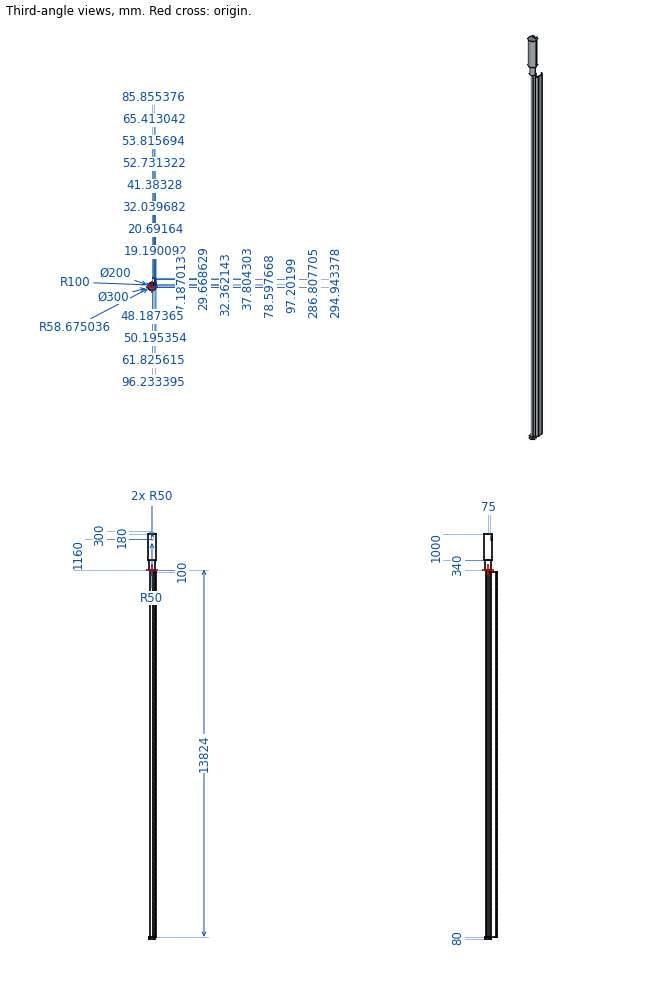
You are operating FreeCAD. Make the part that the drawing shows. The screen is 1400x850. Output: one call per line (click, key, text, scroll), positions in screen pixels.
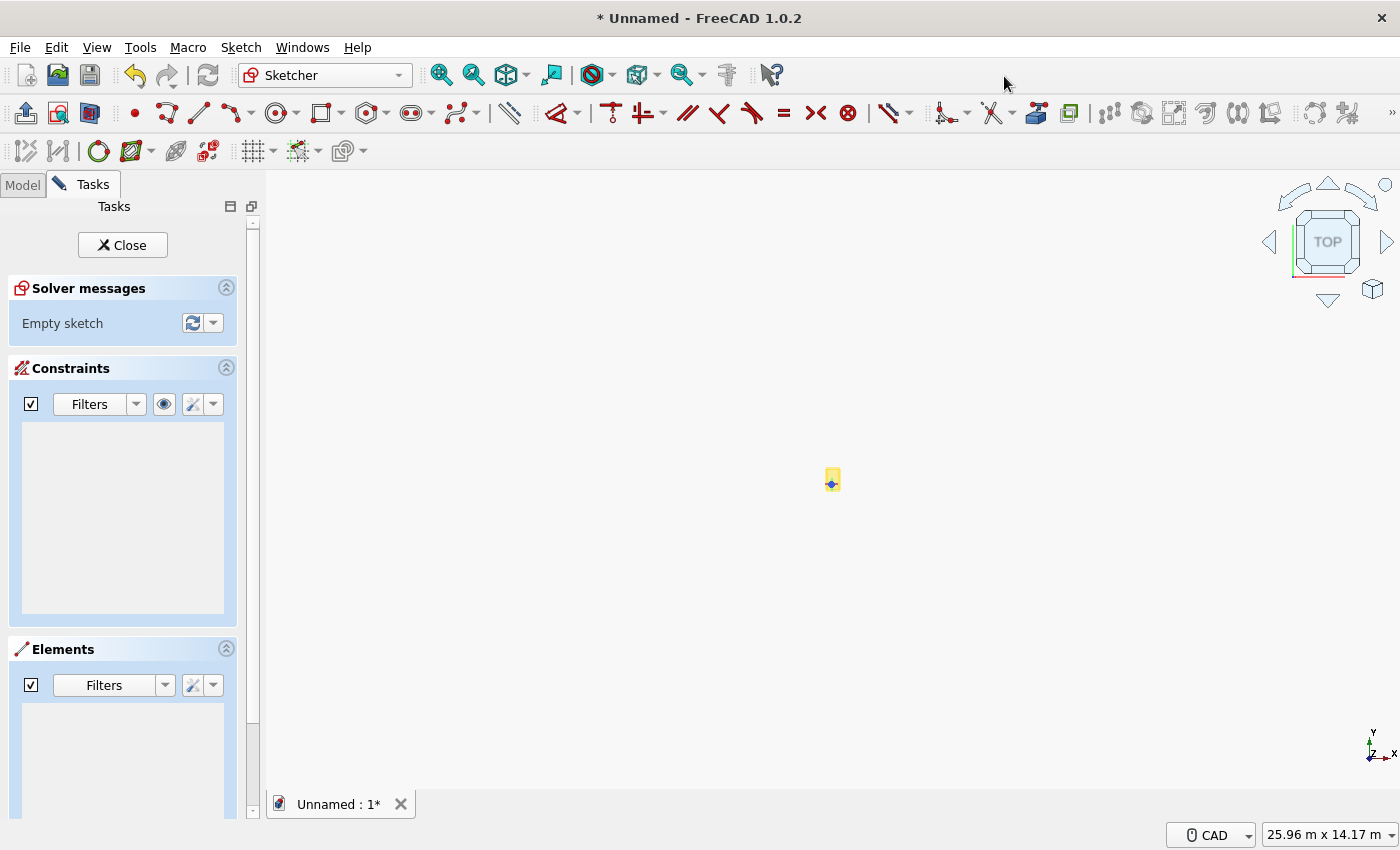
scroll(836, 485, up, 15)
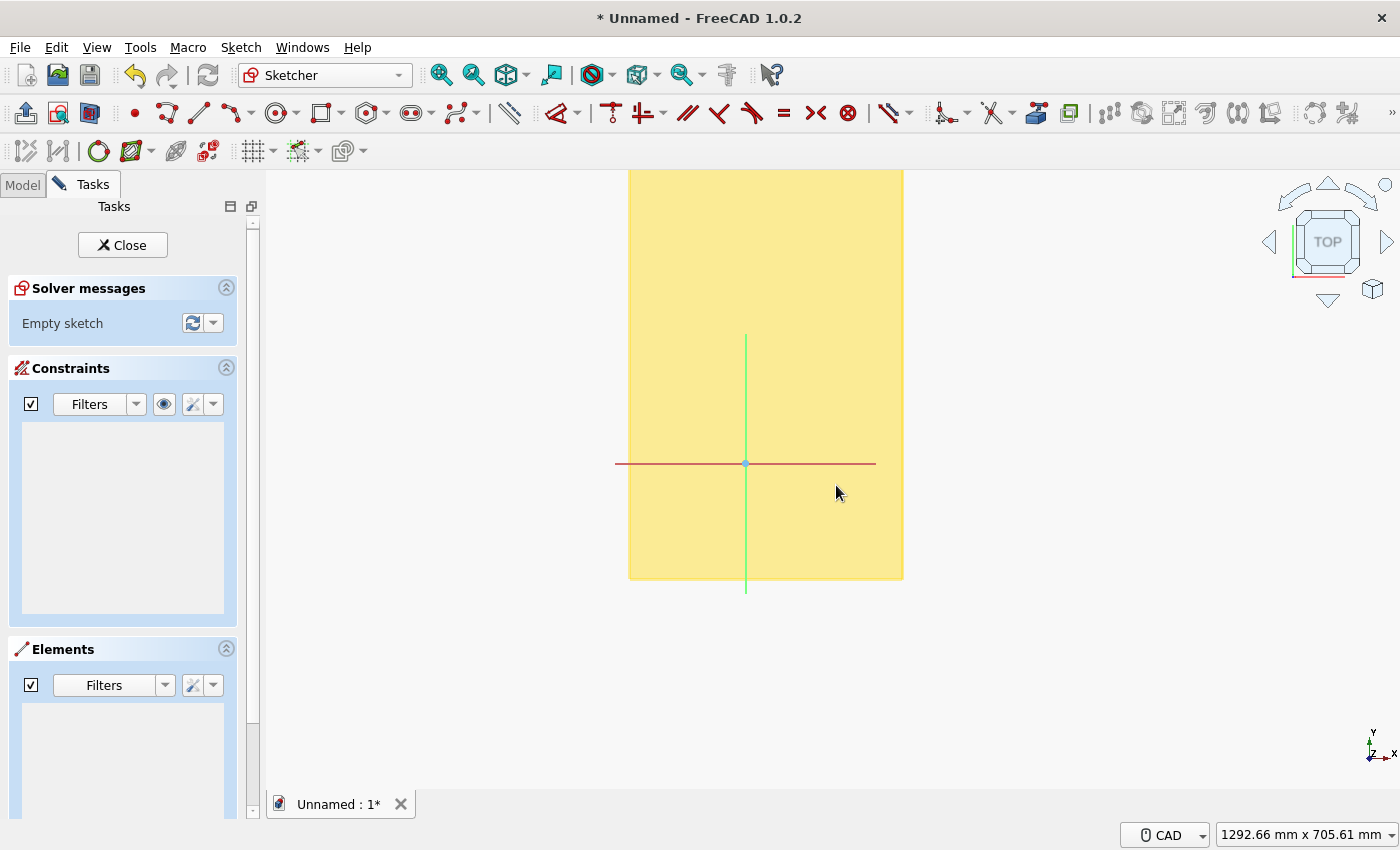
scroll(730, 451, up, 4)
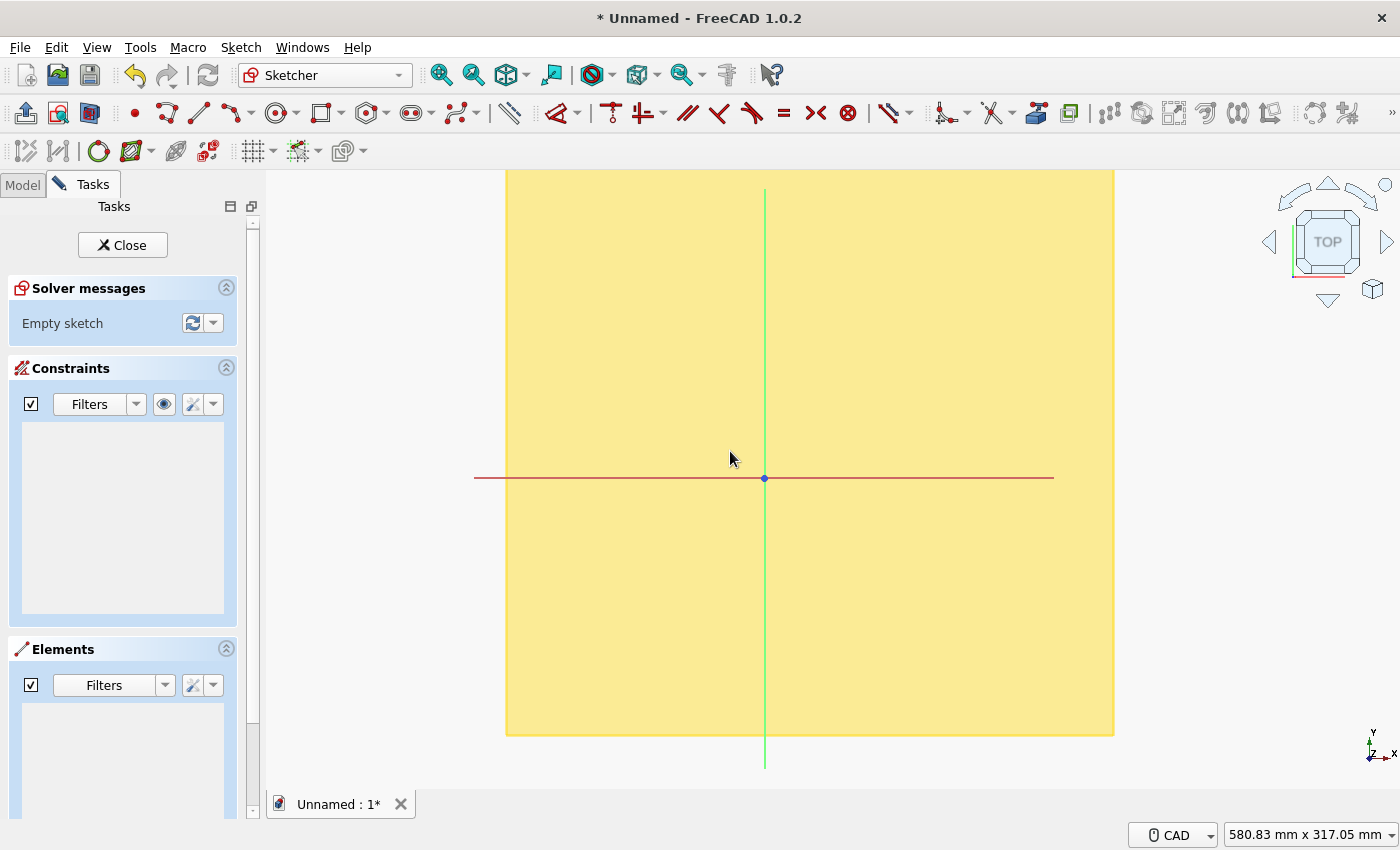
key(g)
key(c)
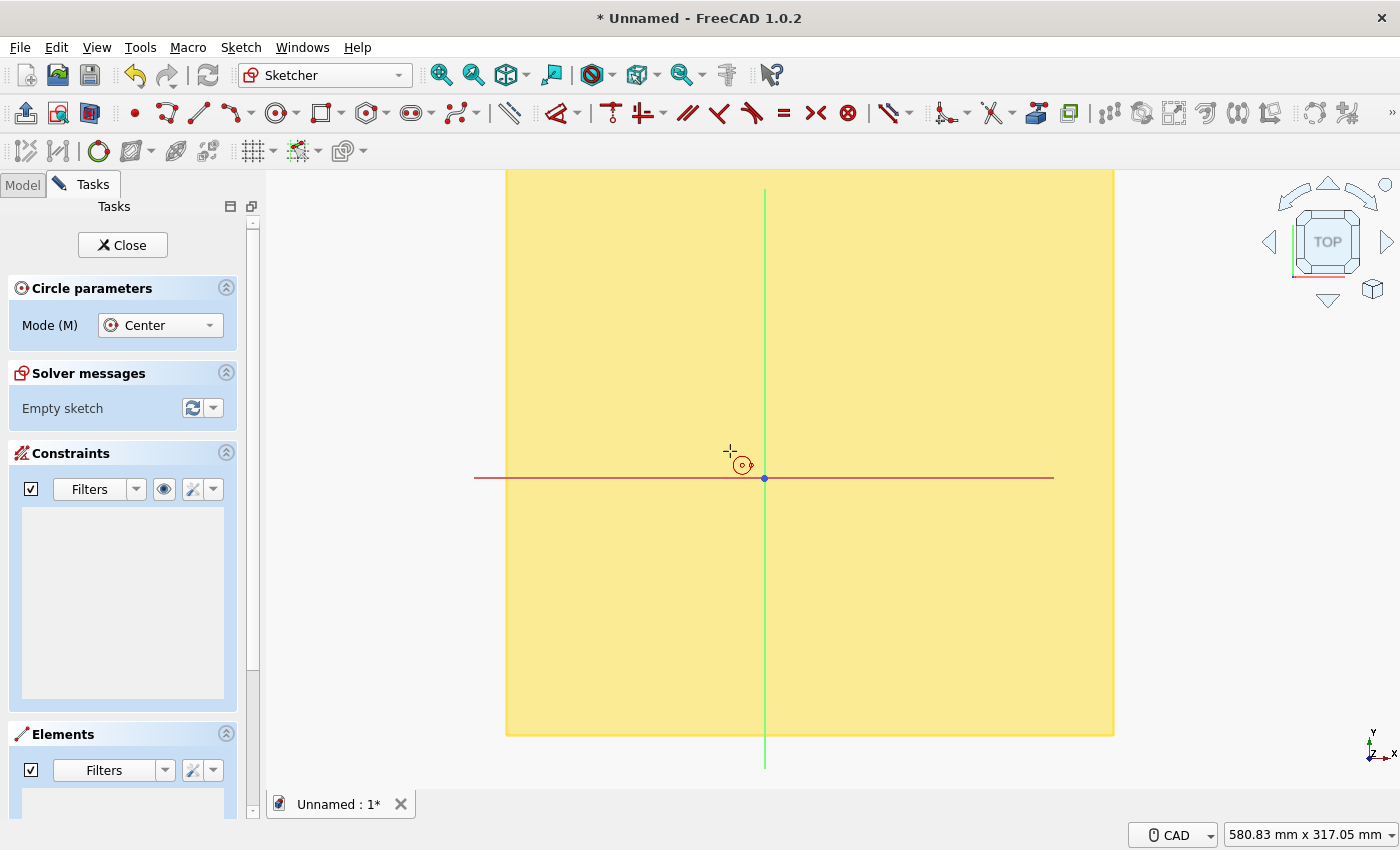
click(765, 478)
click(903, 340)
key(Escape)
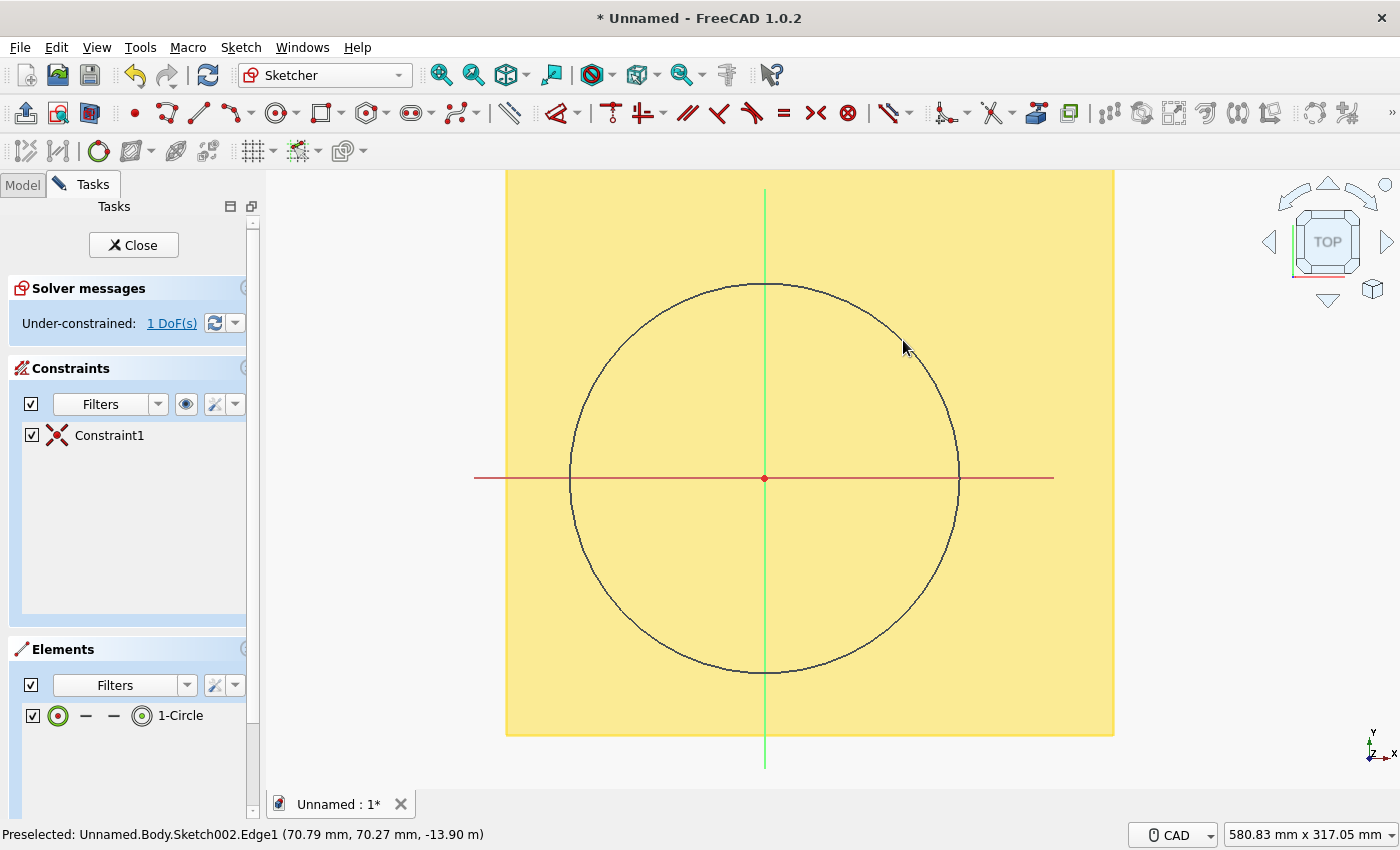
key(d)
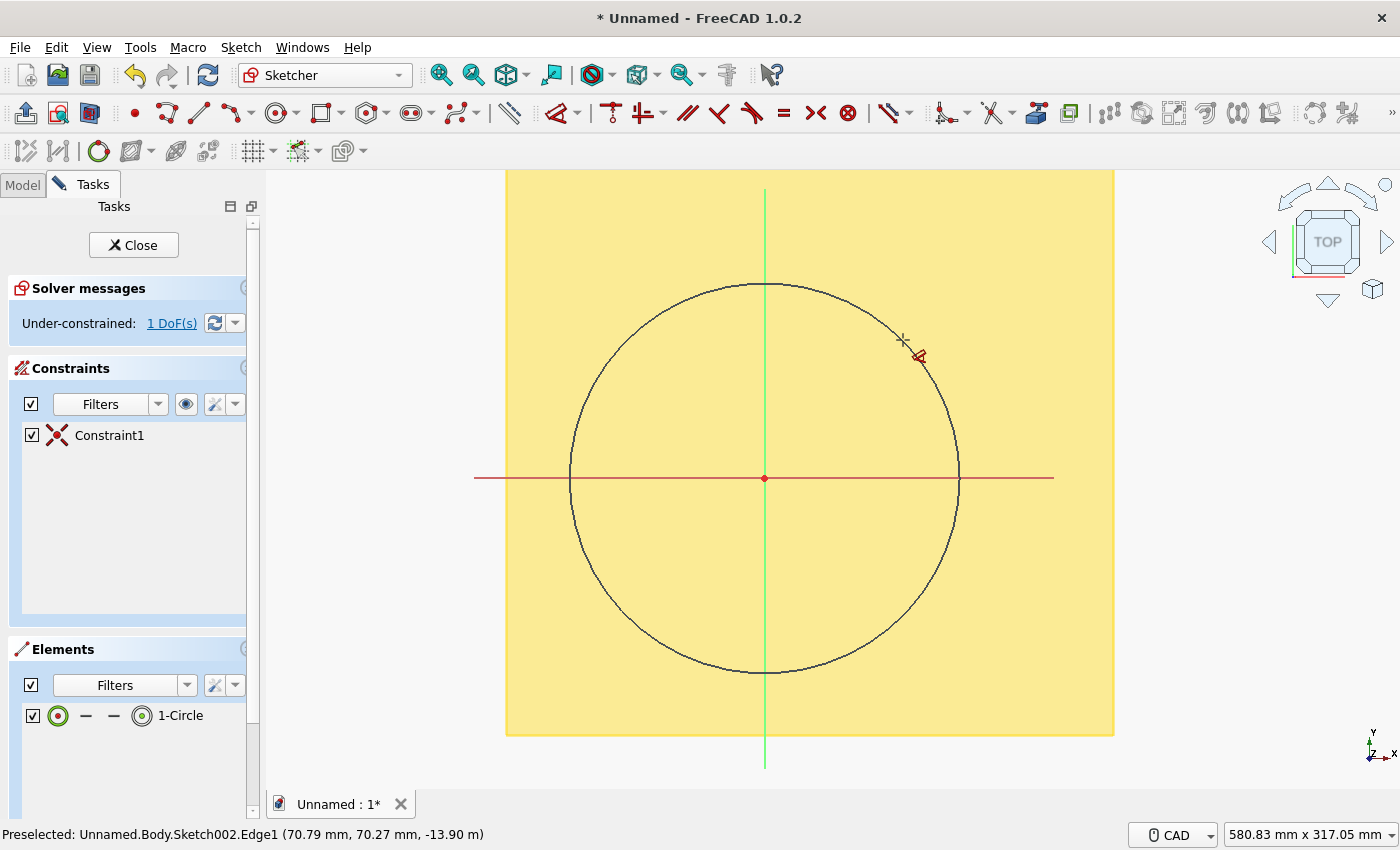
click(902, 340)
click(925, 317)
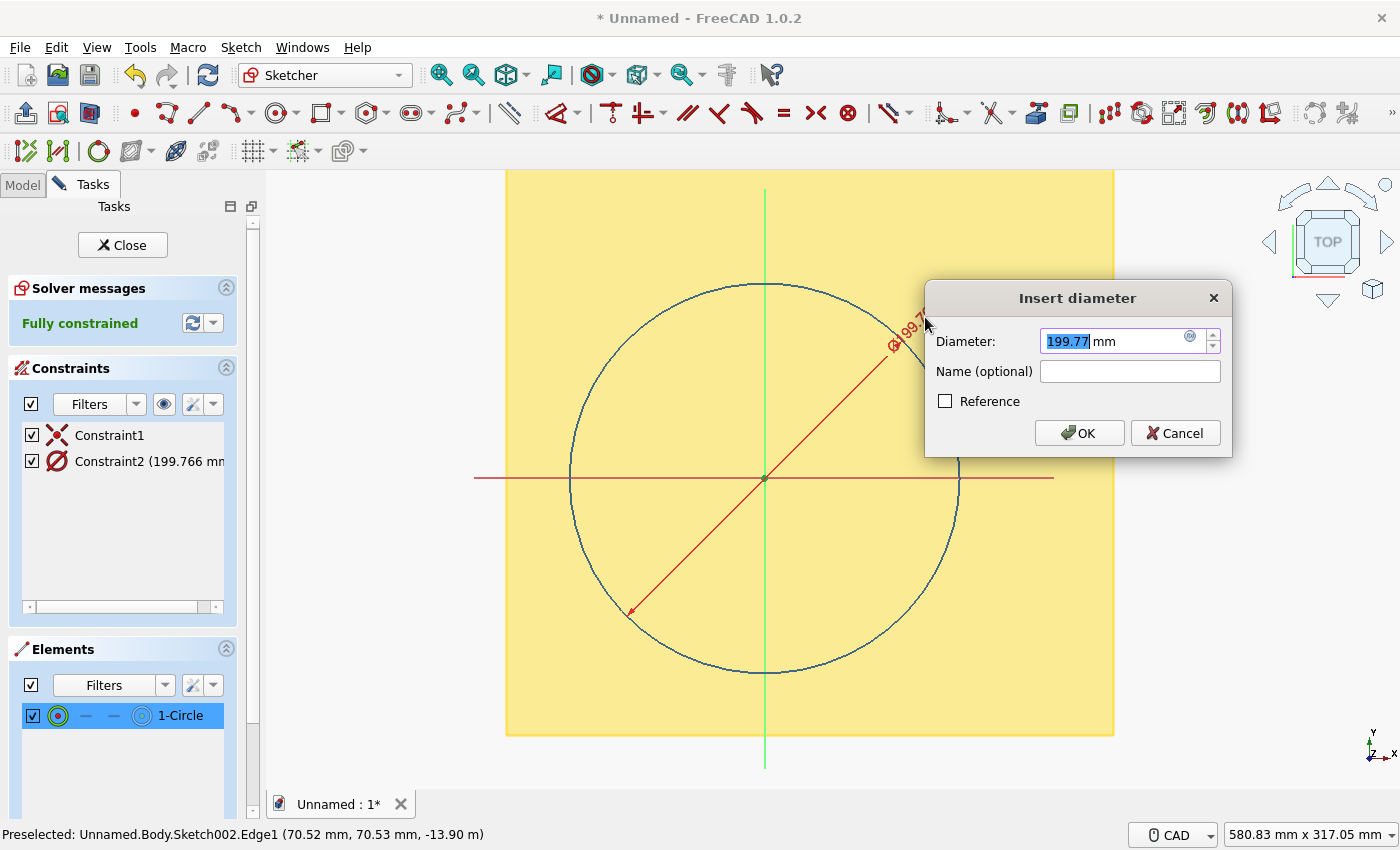
text(200)
key(Return)
key(Escape)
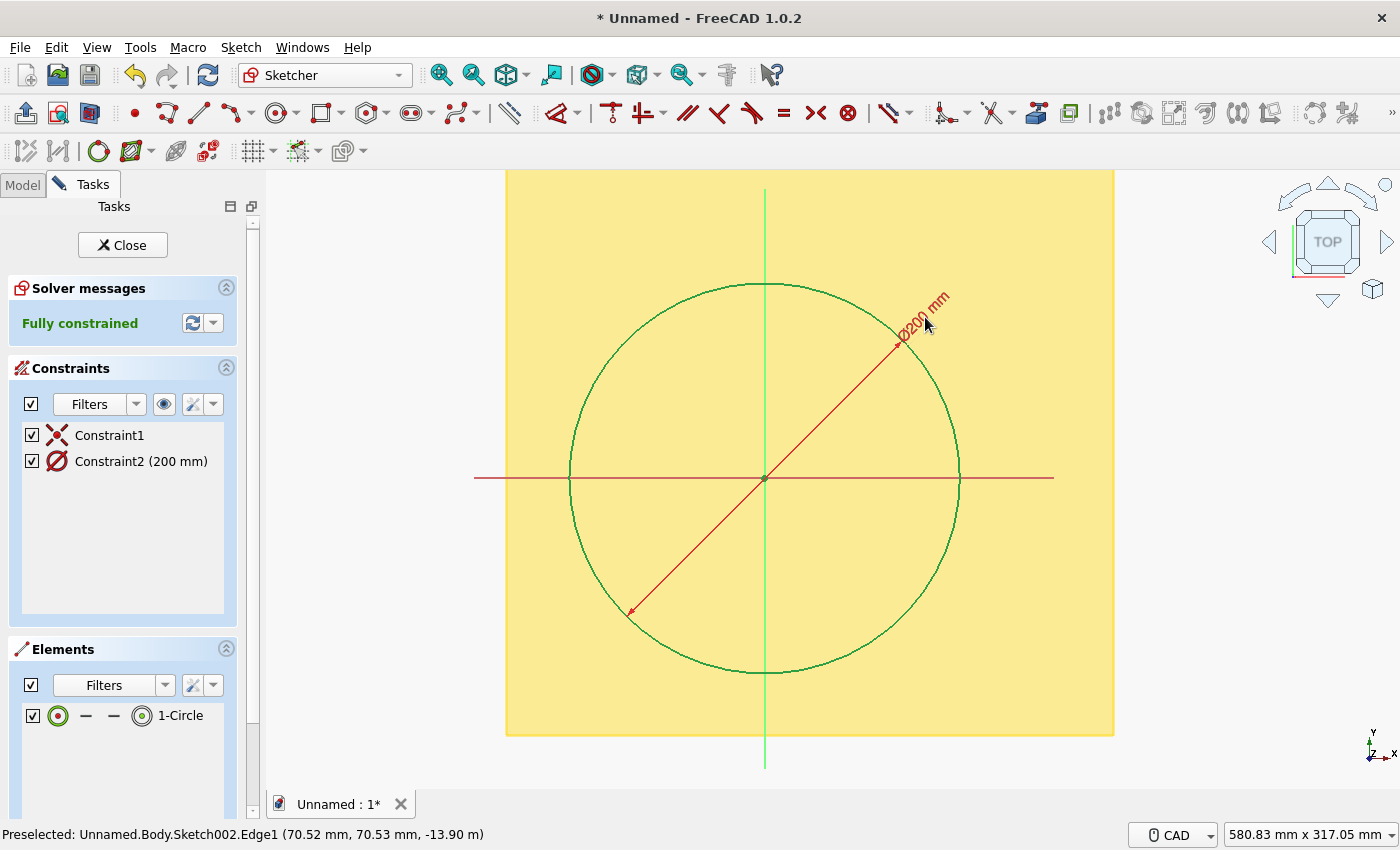
click(123, 245)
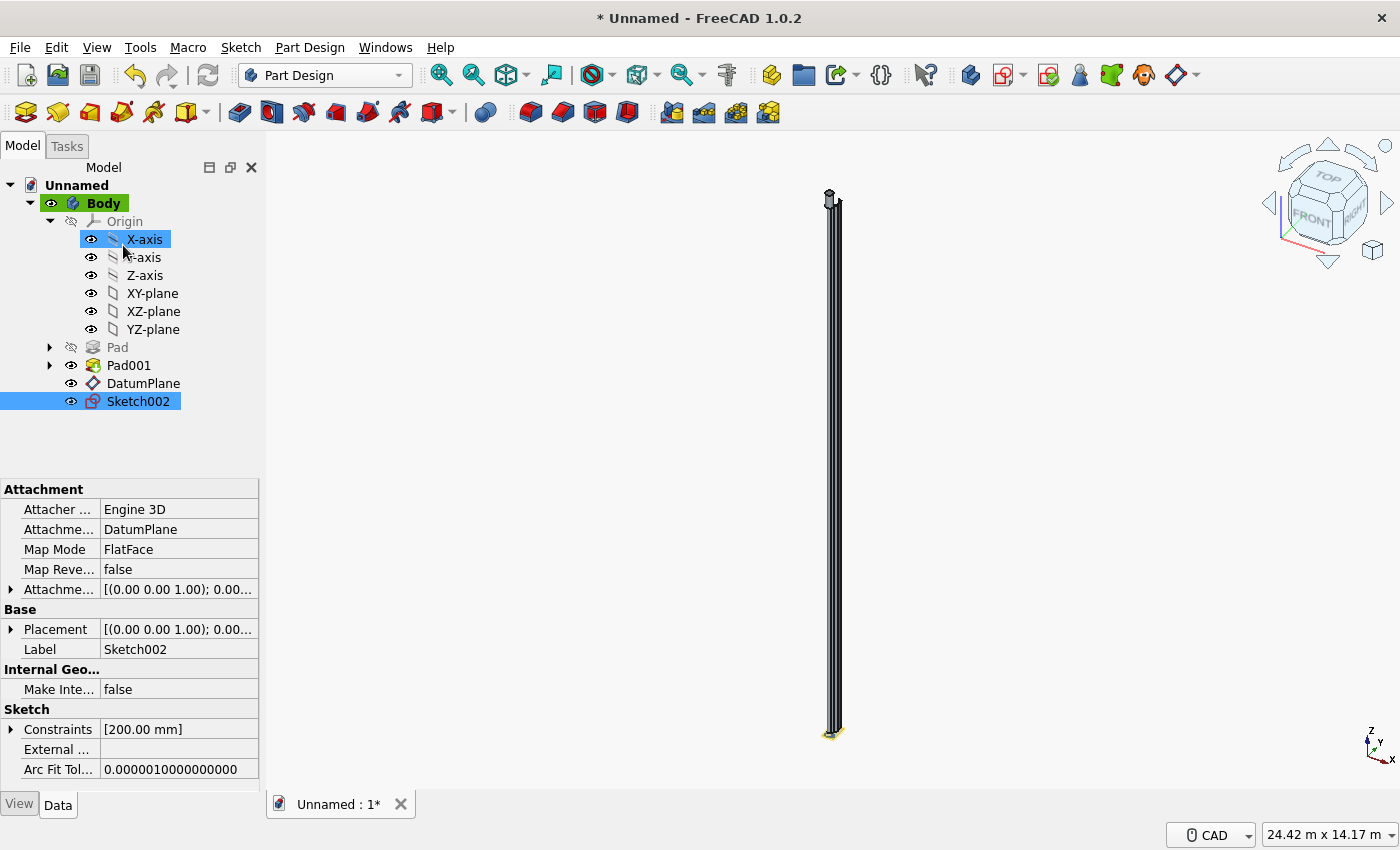
click(26, 112)